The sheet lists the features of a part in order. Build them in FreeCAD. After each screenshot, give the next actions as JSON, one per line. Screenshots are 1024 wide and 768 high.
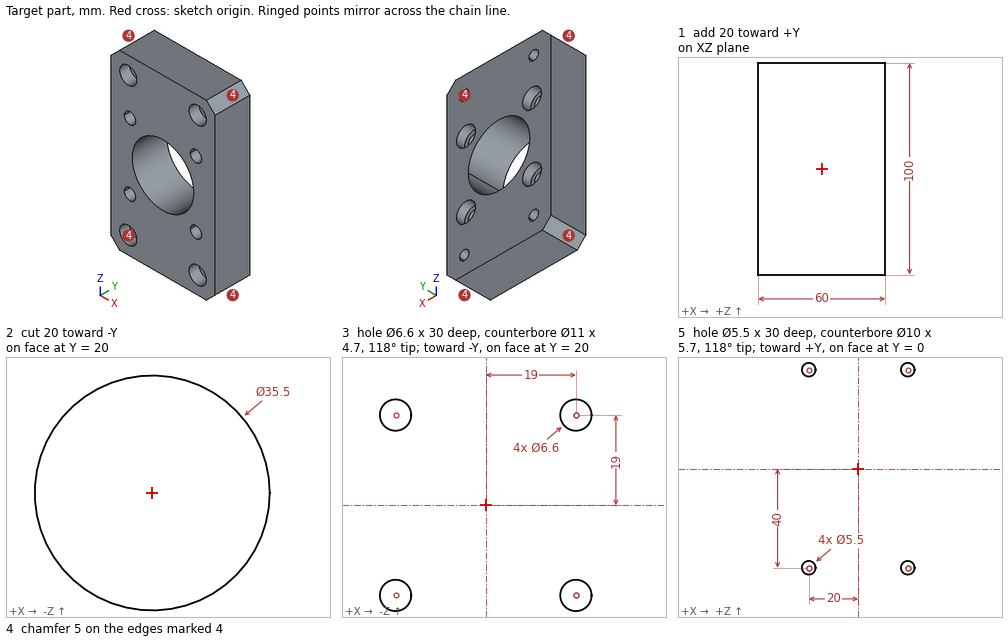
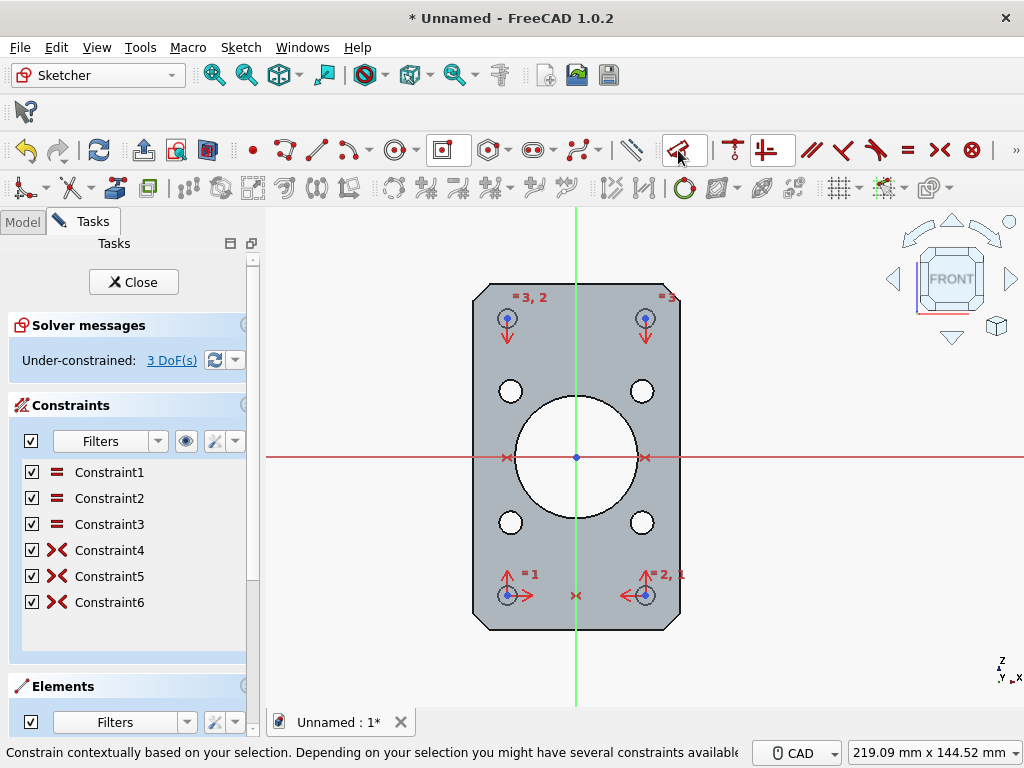
{"action": "scroll", "coordinate": [514, 589], "scroll_direction": "up", "scroll_amount": 4}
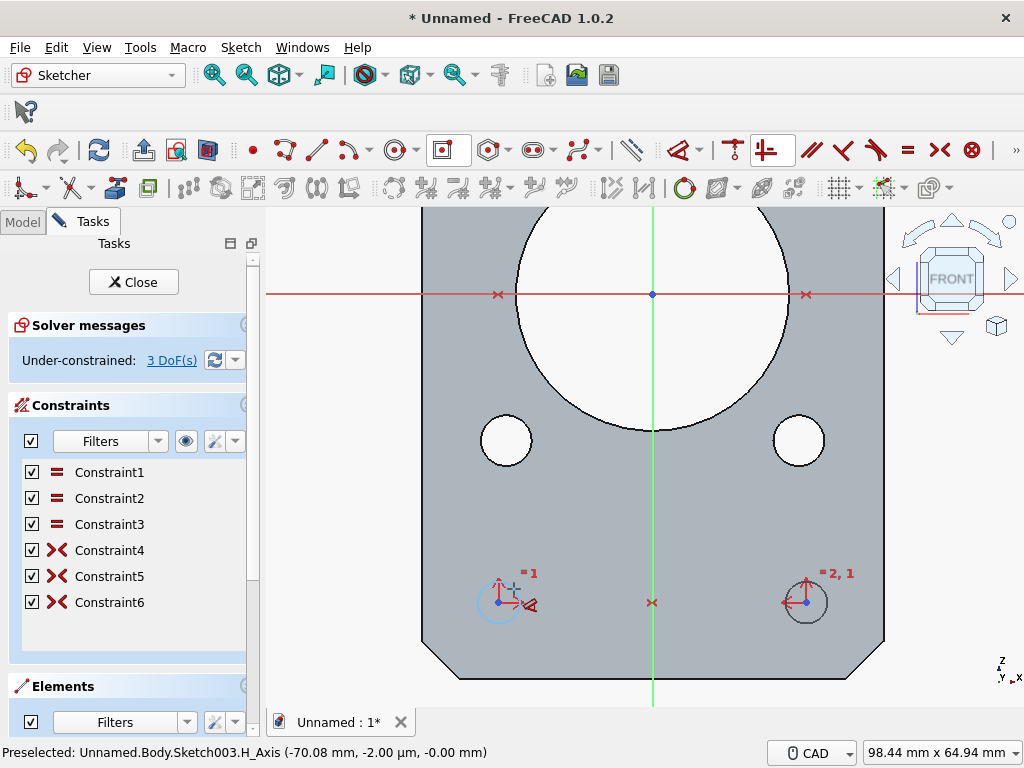
{"action": "left_click", "coordinate": [514, 588]}
{"action": "left_click", "coordinate": [537, 566]}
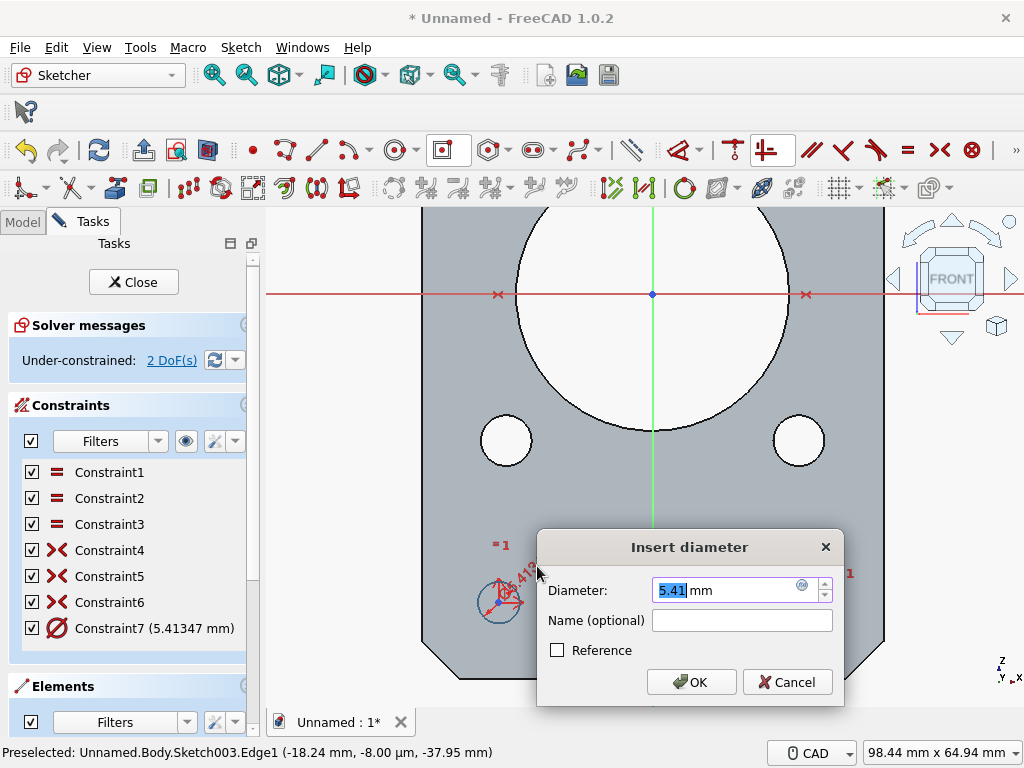
{"action": "type", "text": "5.5"}
{"action": "key", "text": "Return"}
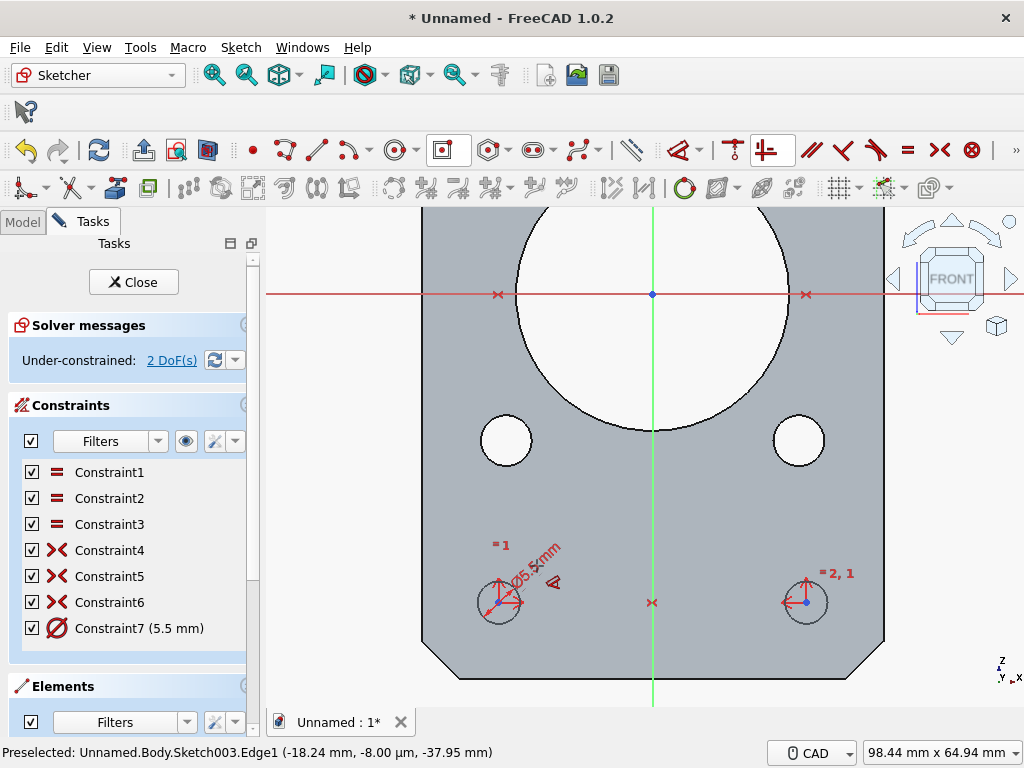
{"action": "left_click", "coordinate": [499, 603]}
{"action": "left_click", "coordinate": [576, 637]}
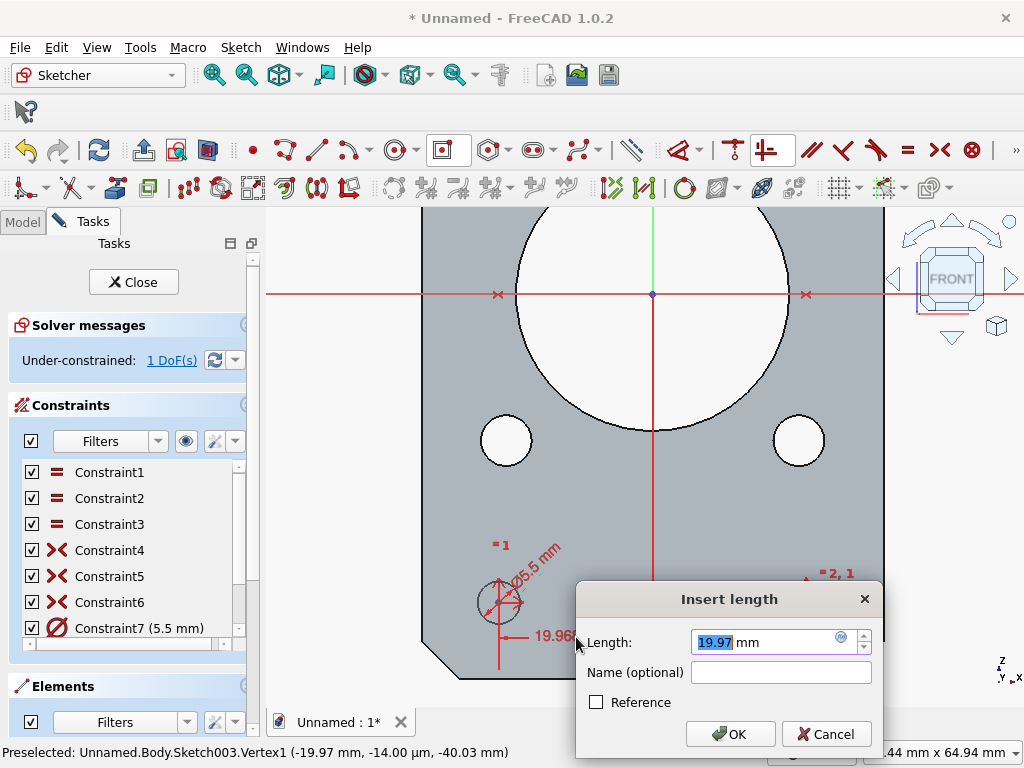
{"action": "type", "text": "20"}
{"action": "key", "text": "Return"}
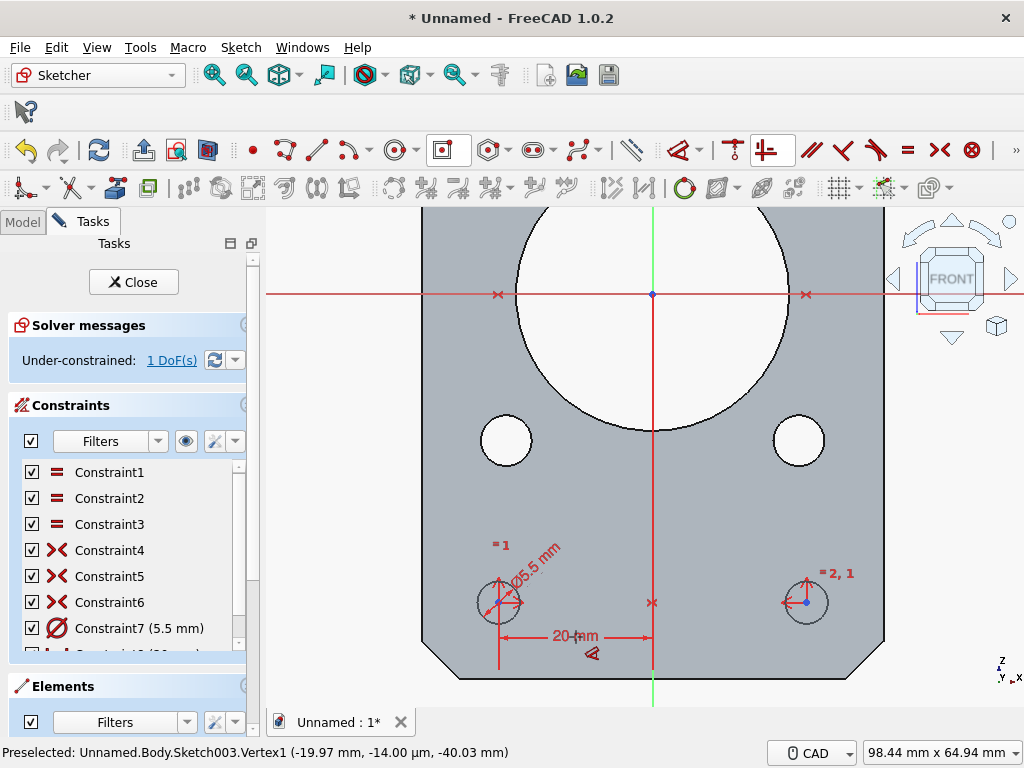
{"action": "left_click", "coordinate": [499, 603]}
{"action": "left_click", "coordinate": [465, 449]}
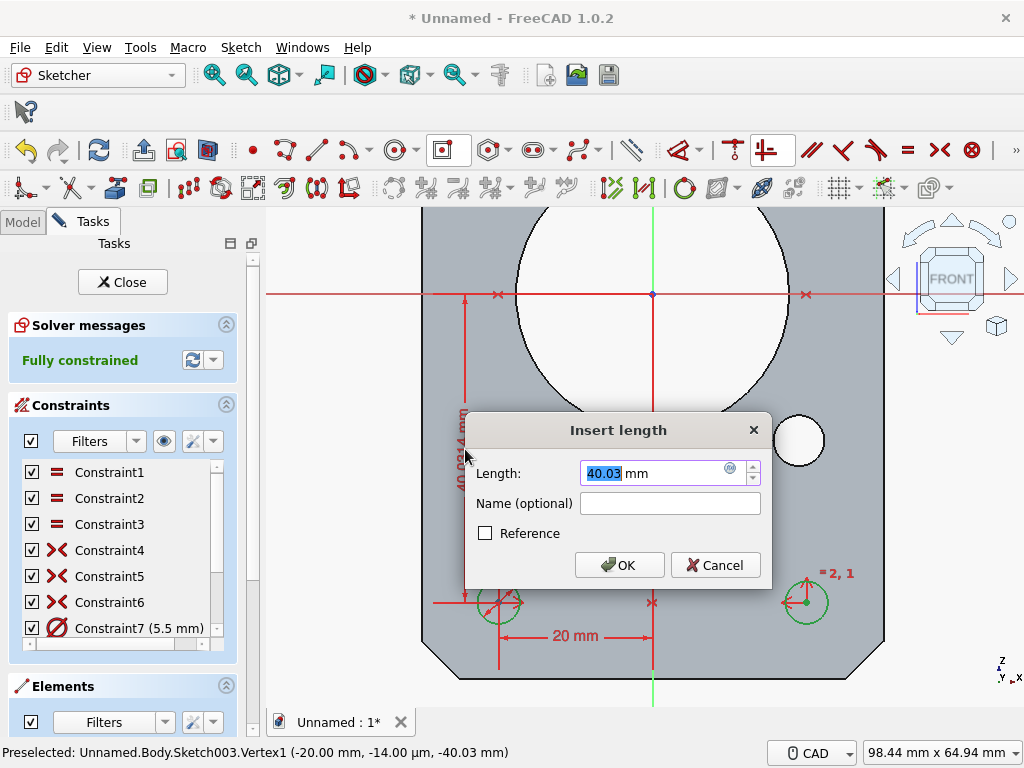
{"action": "type", "text": "40"}
{"action": "key", "text": "Return"}
{"action": "key", "text": "Escape"}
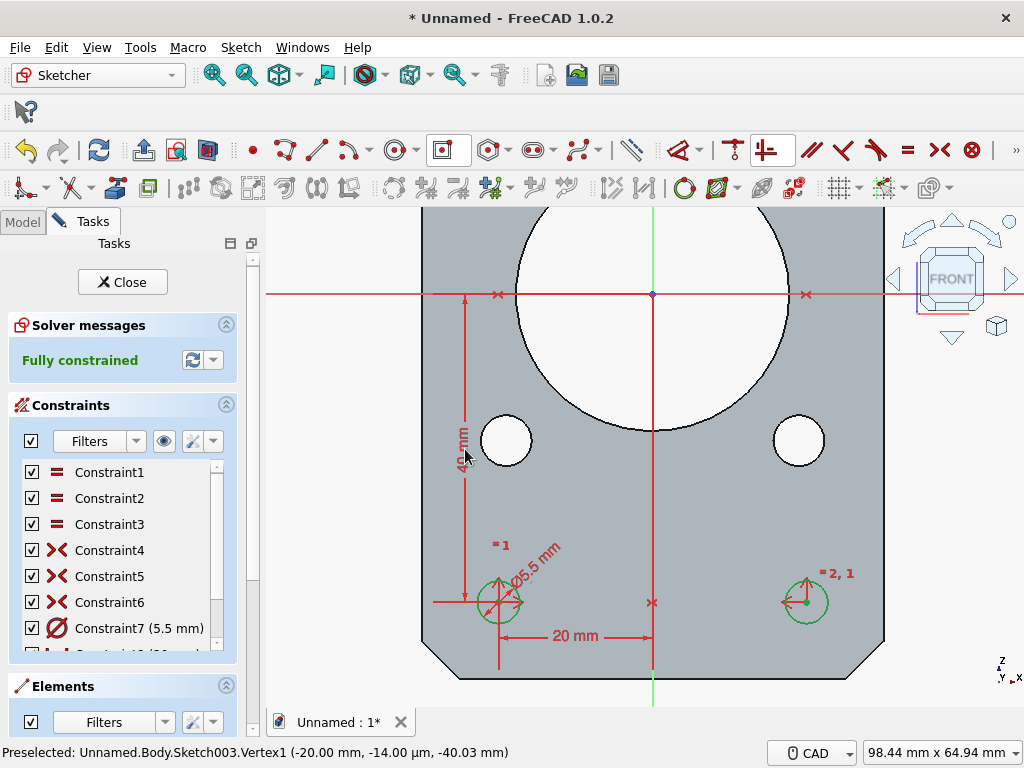
{"action": "left_click", "coordinate": [123, 282]}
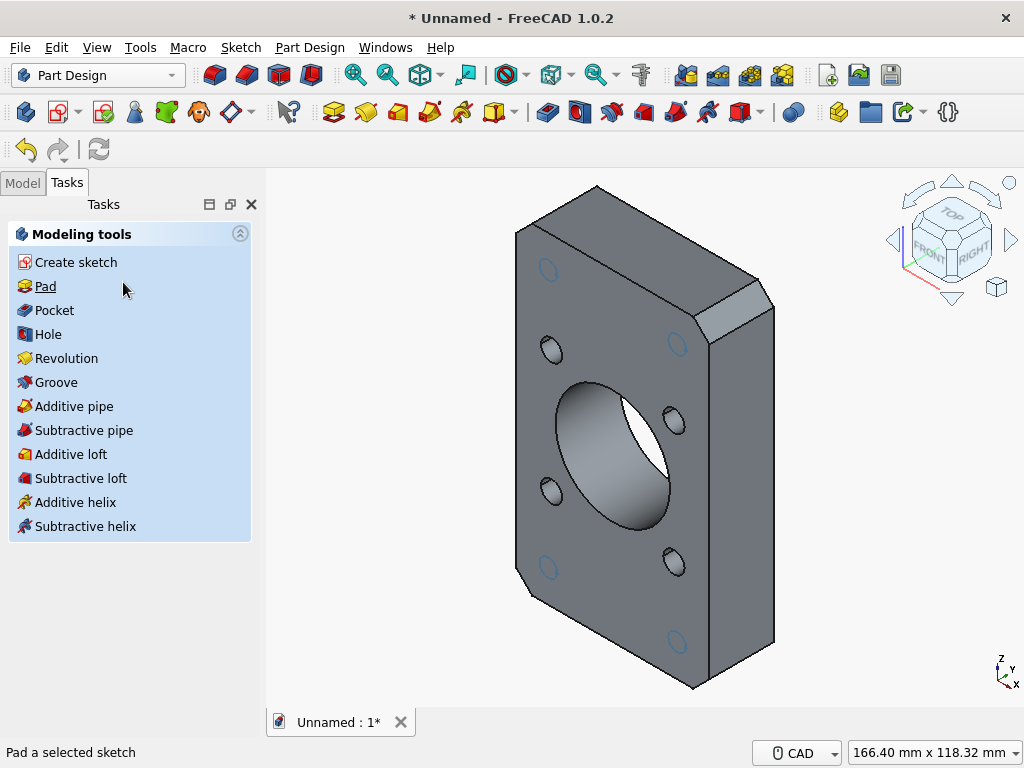
{"action": "left_click", "coordinate": [580, 112]}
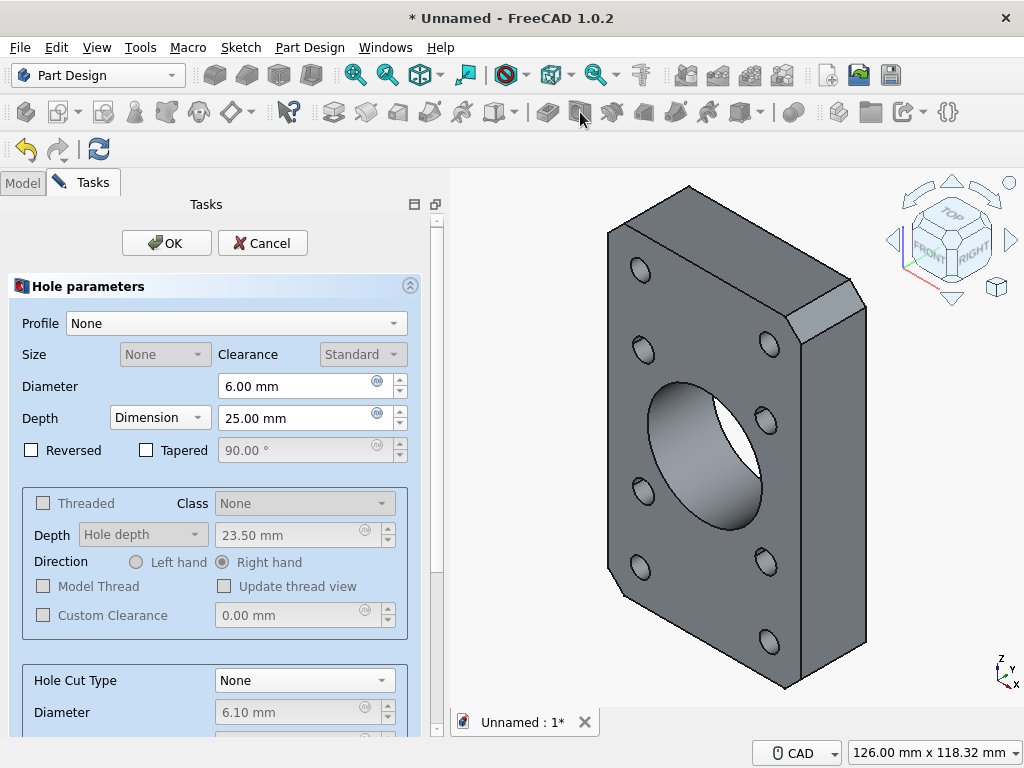
{"action": "triple_click", "coordinate": [305, 386]}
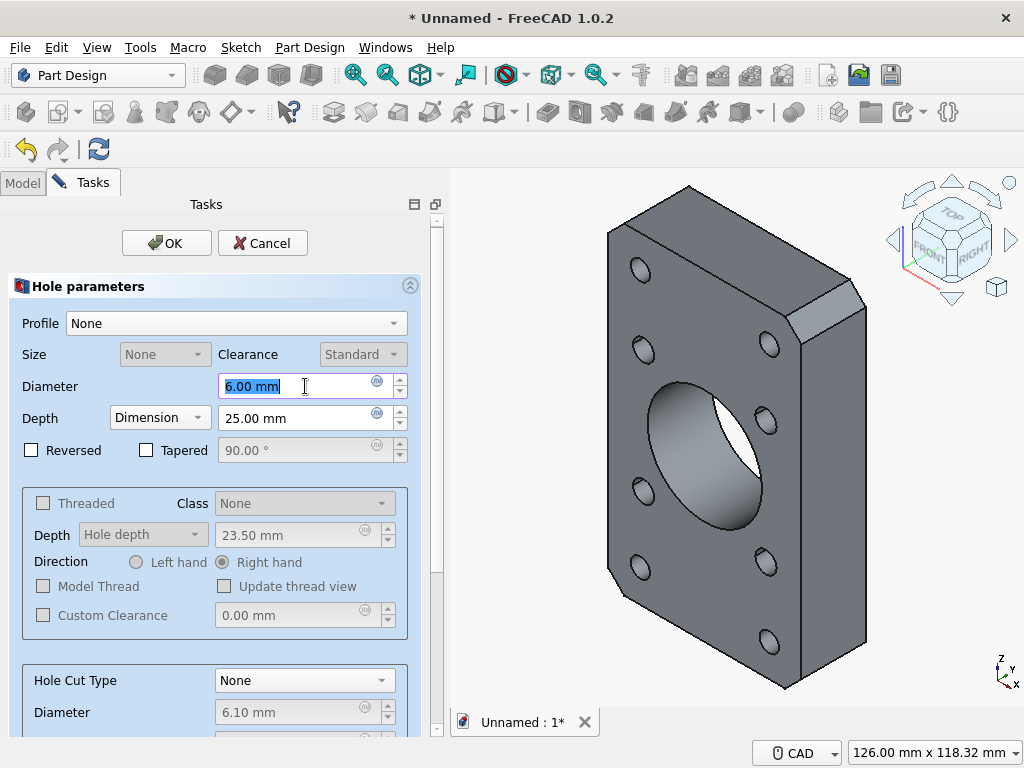
{"action": "type", "text": "5.5"}
{"action": "key", "text": "Tab"}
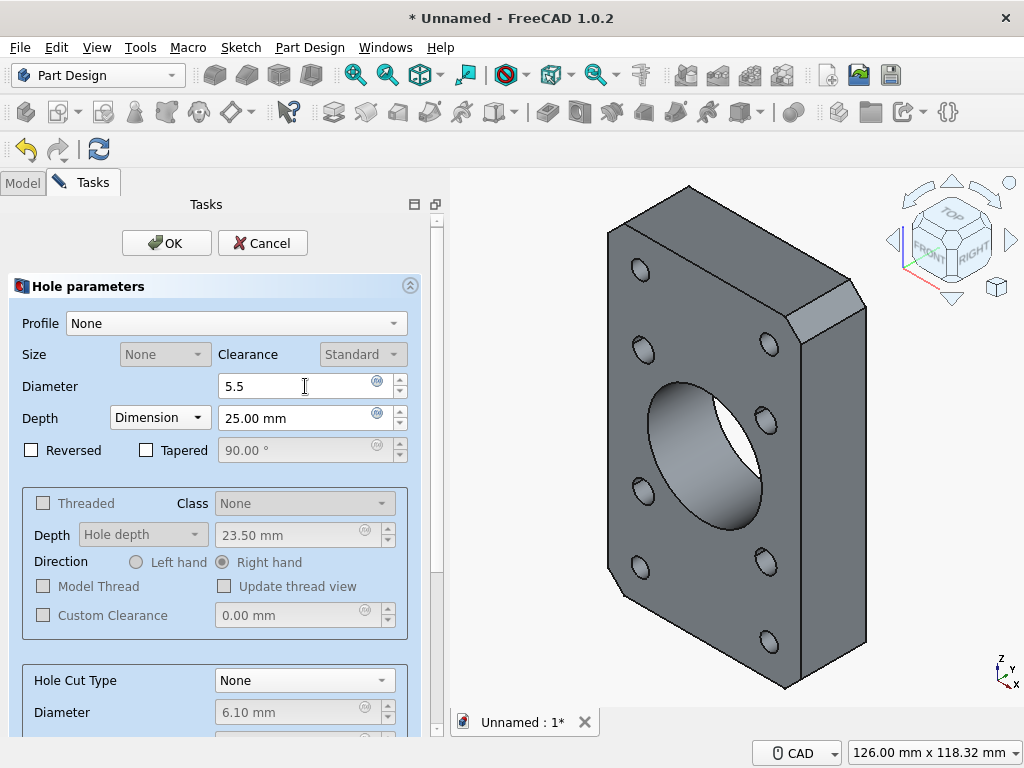
{"action": "triple_click", "coordinate": [305, 418]}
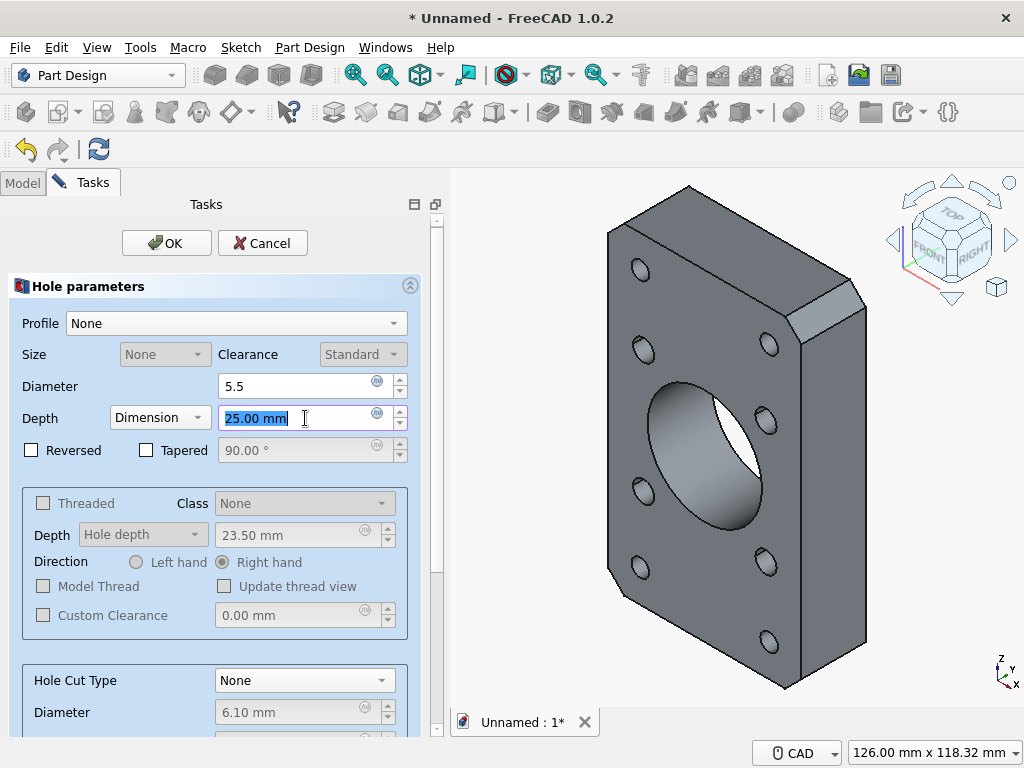
{"action": "type", "text": "30"}
{"action": "key", "text": "Tab"}